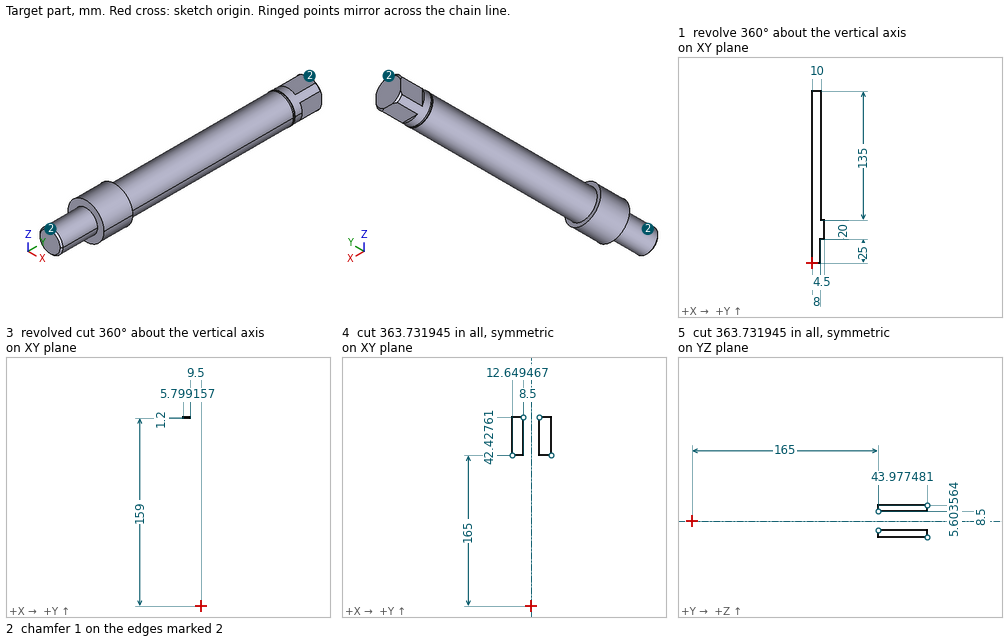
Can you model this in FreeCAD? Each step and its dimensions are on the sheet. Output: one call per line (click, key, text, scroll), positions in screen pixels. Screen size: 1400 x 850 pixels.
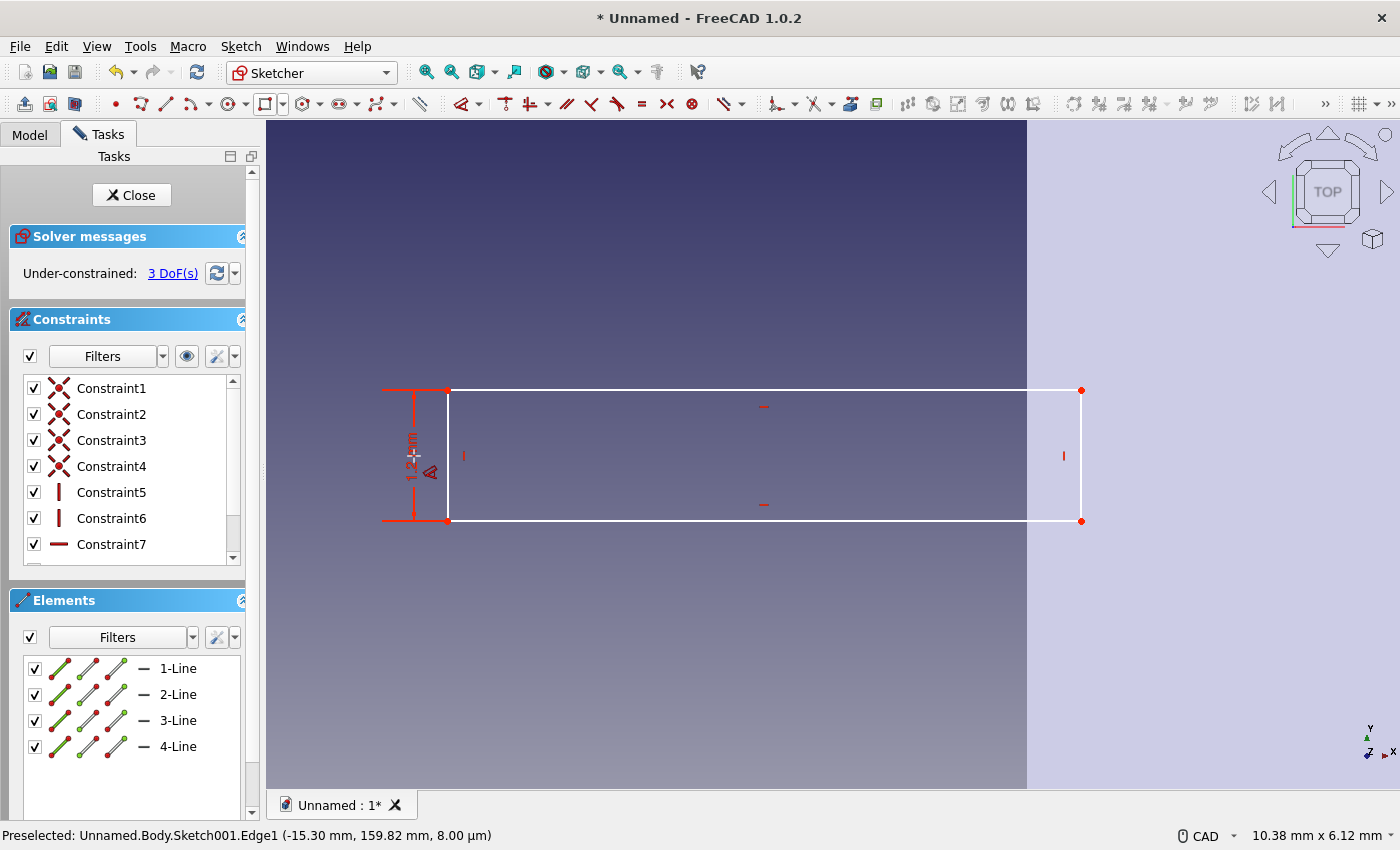
click(448, 521)
click(414, 641)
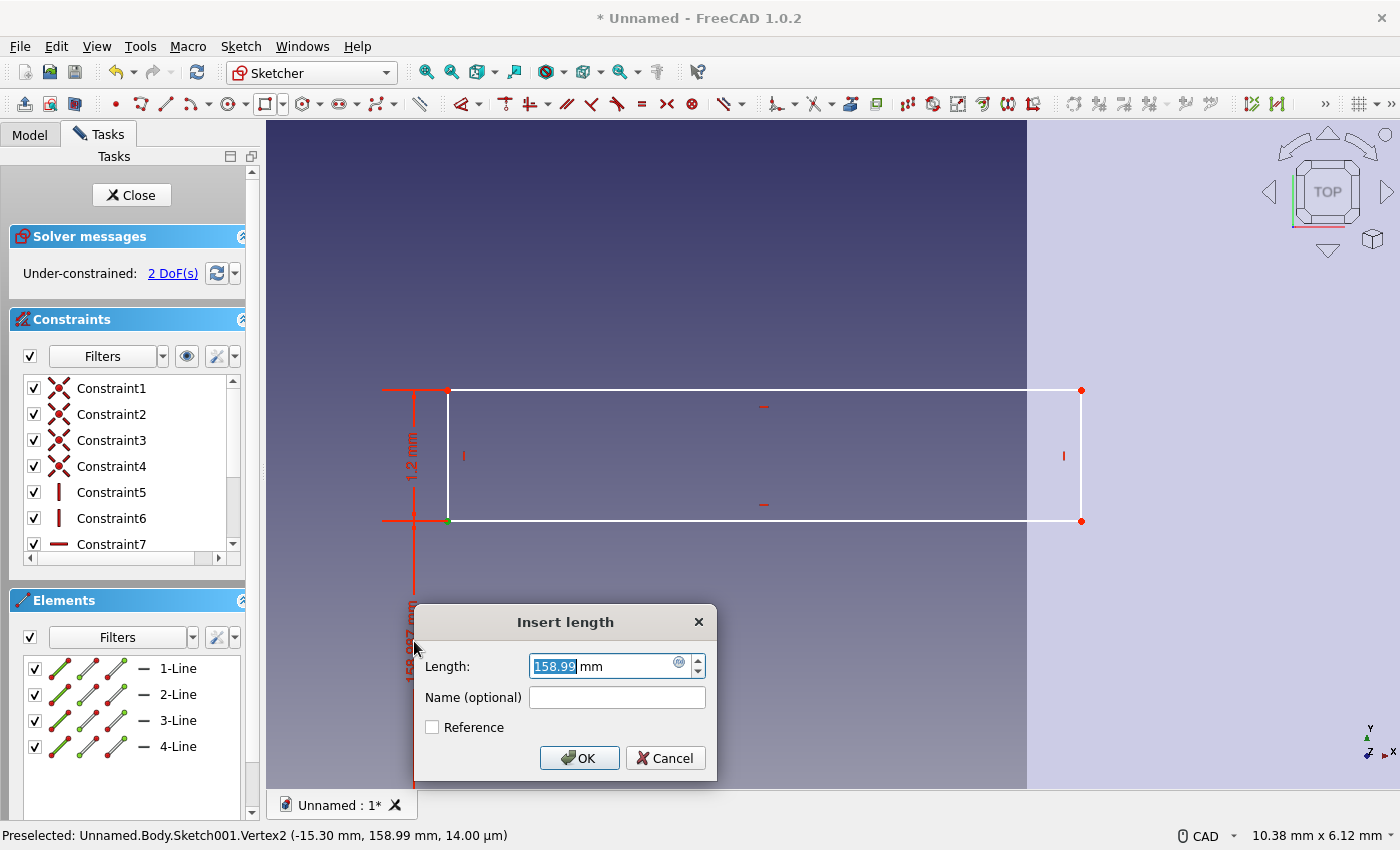
text(159)
key(Return)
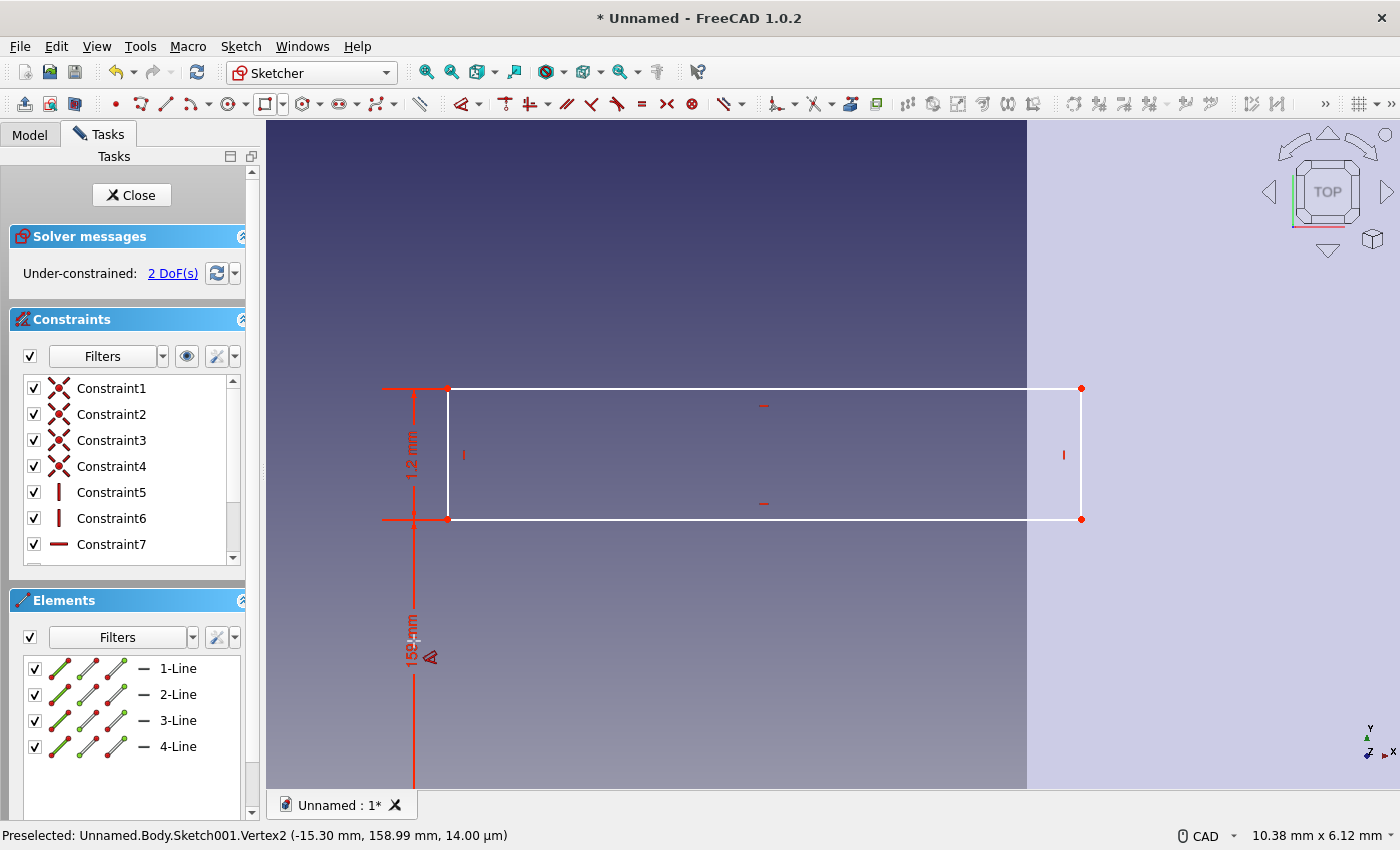
click(1081, 520)
click(1158, 486)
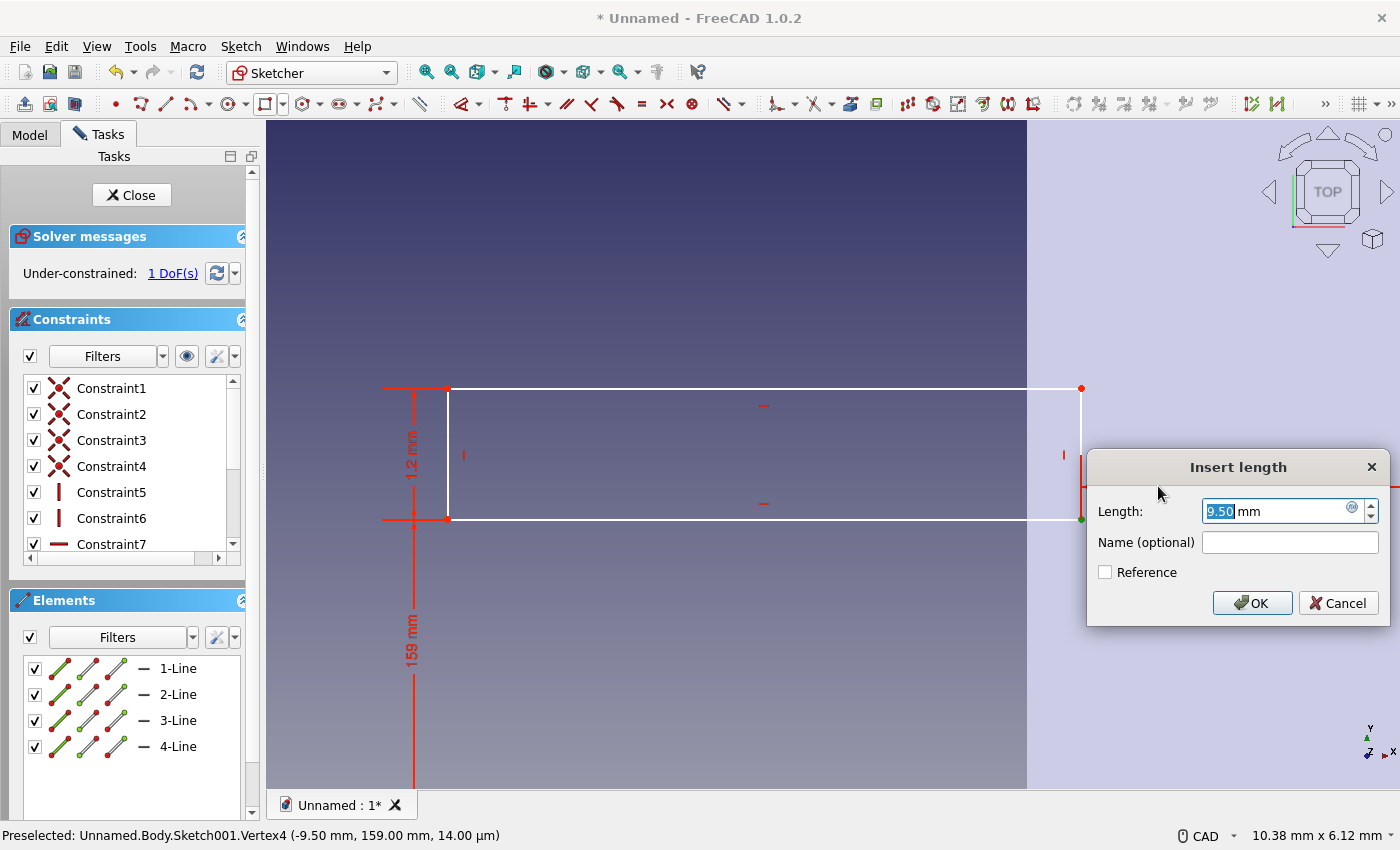
text(9.5)
key(Return)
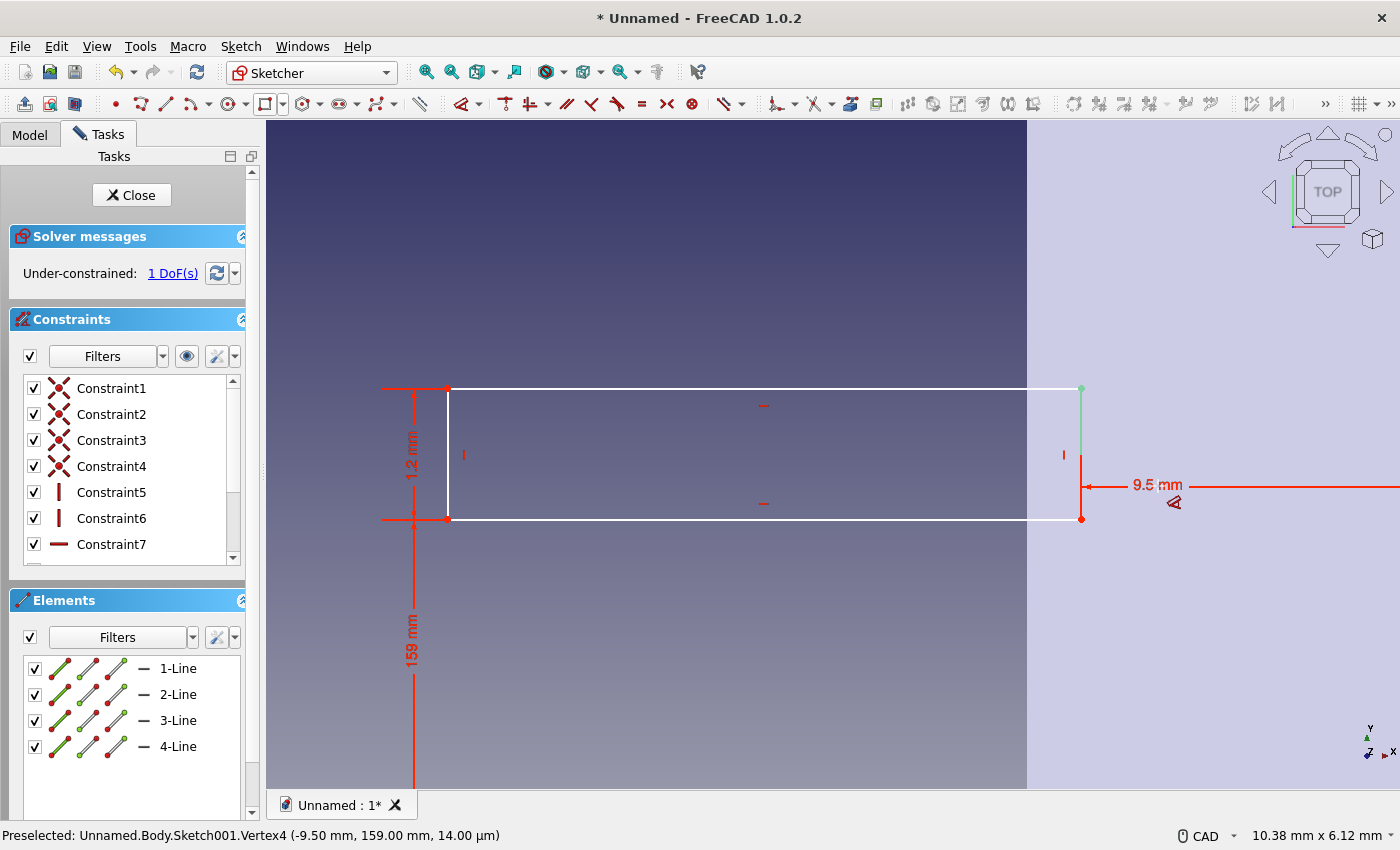
click(638, 520)
click(765, 554)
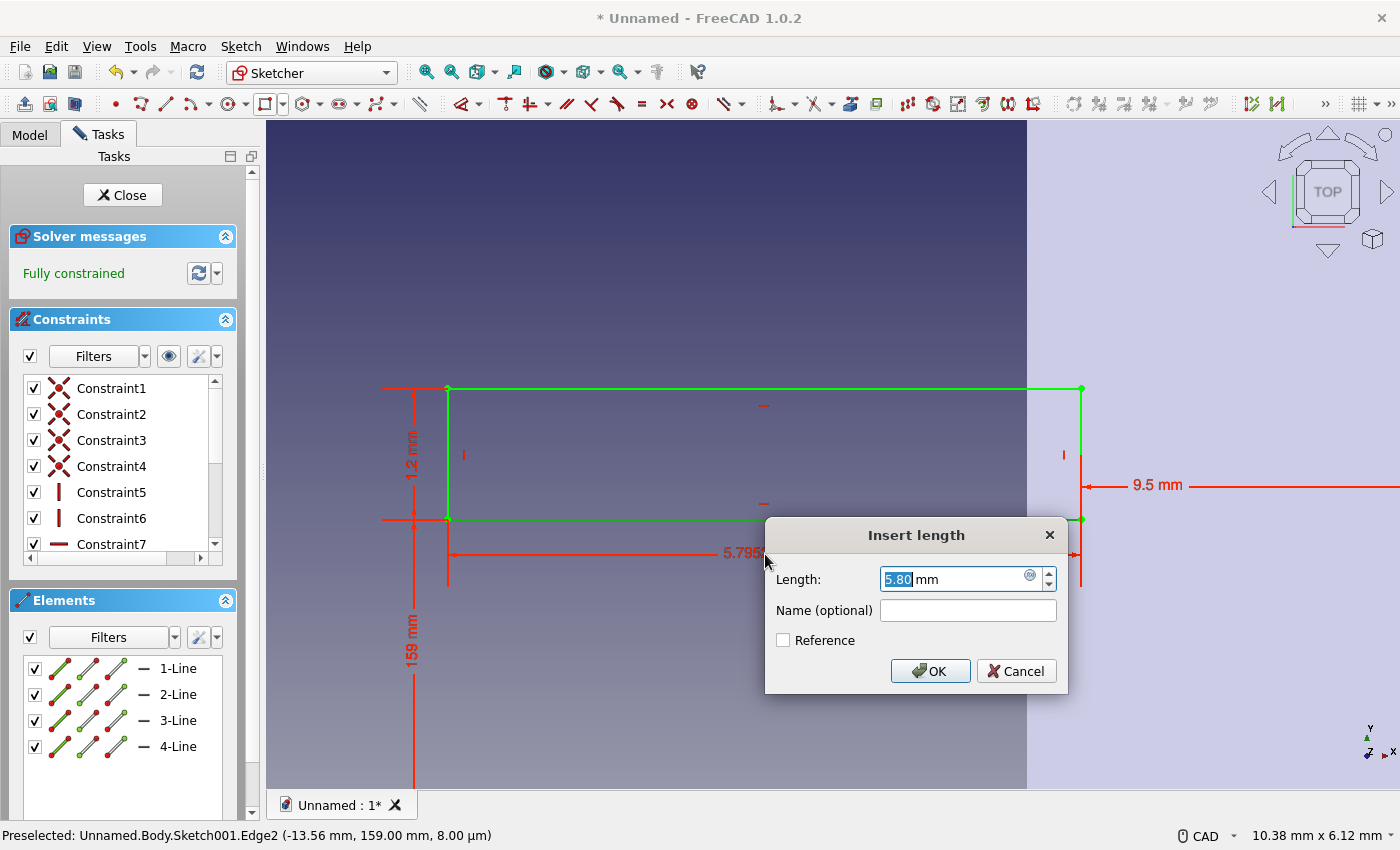
text(5.799157)
key(Return)
key(Escape)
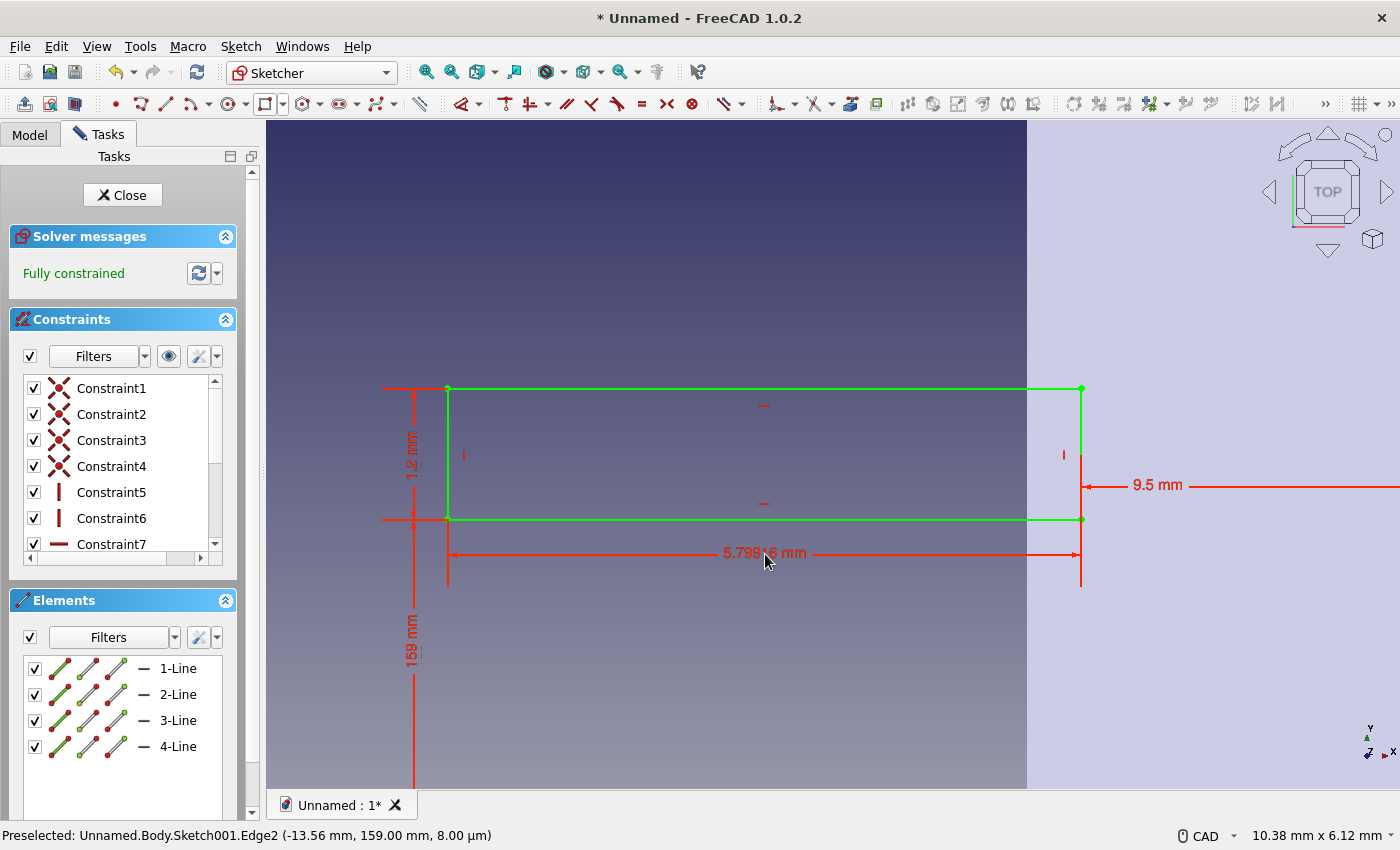
click(123, 195)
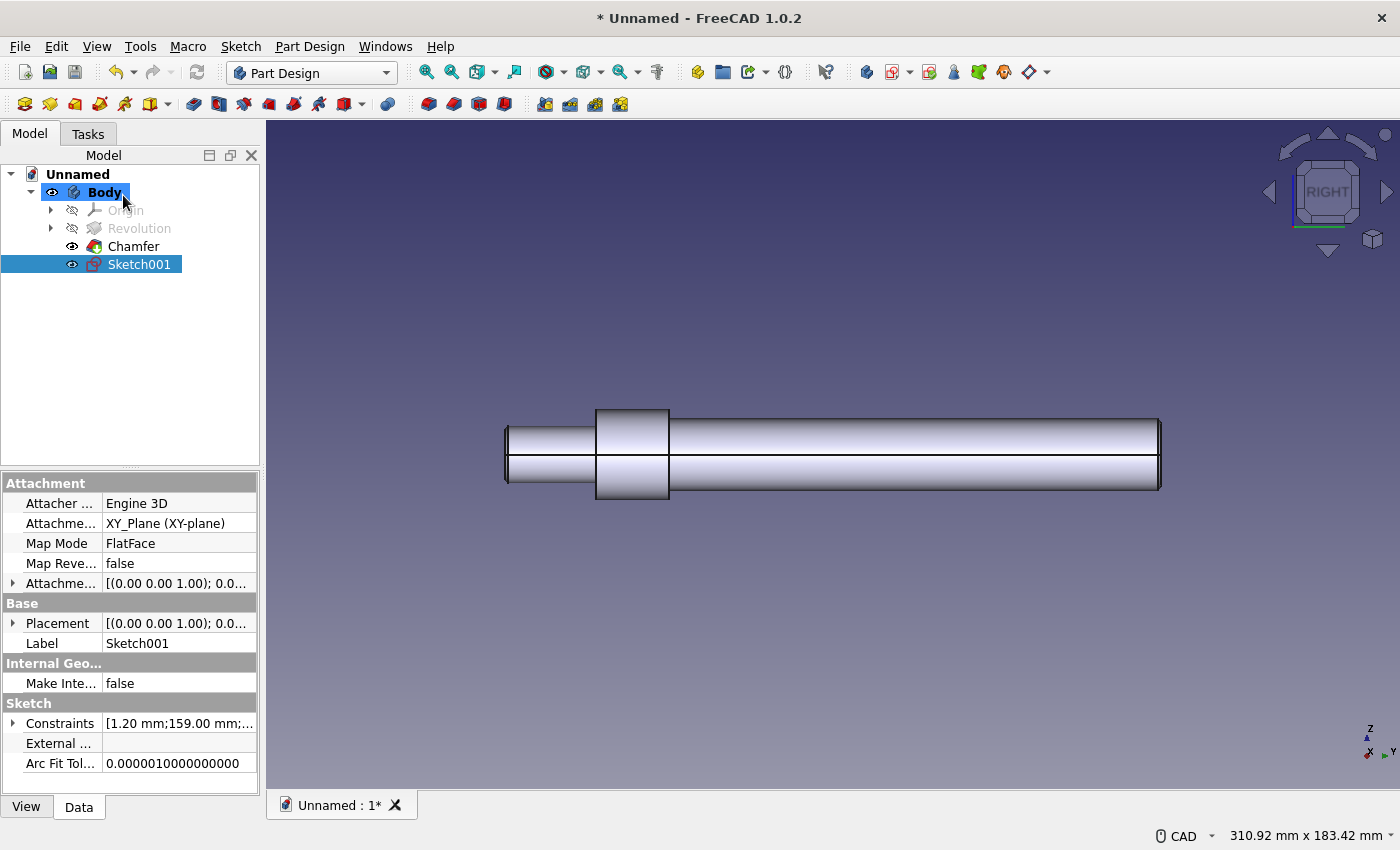
click(244, 104)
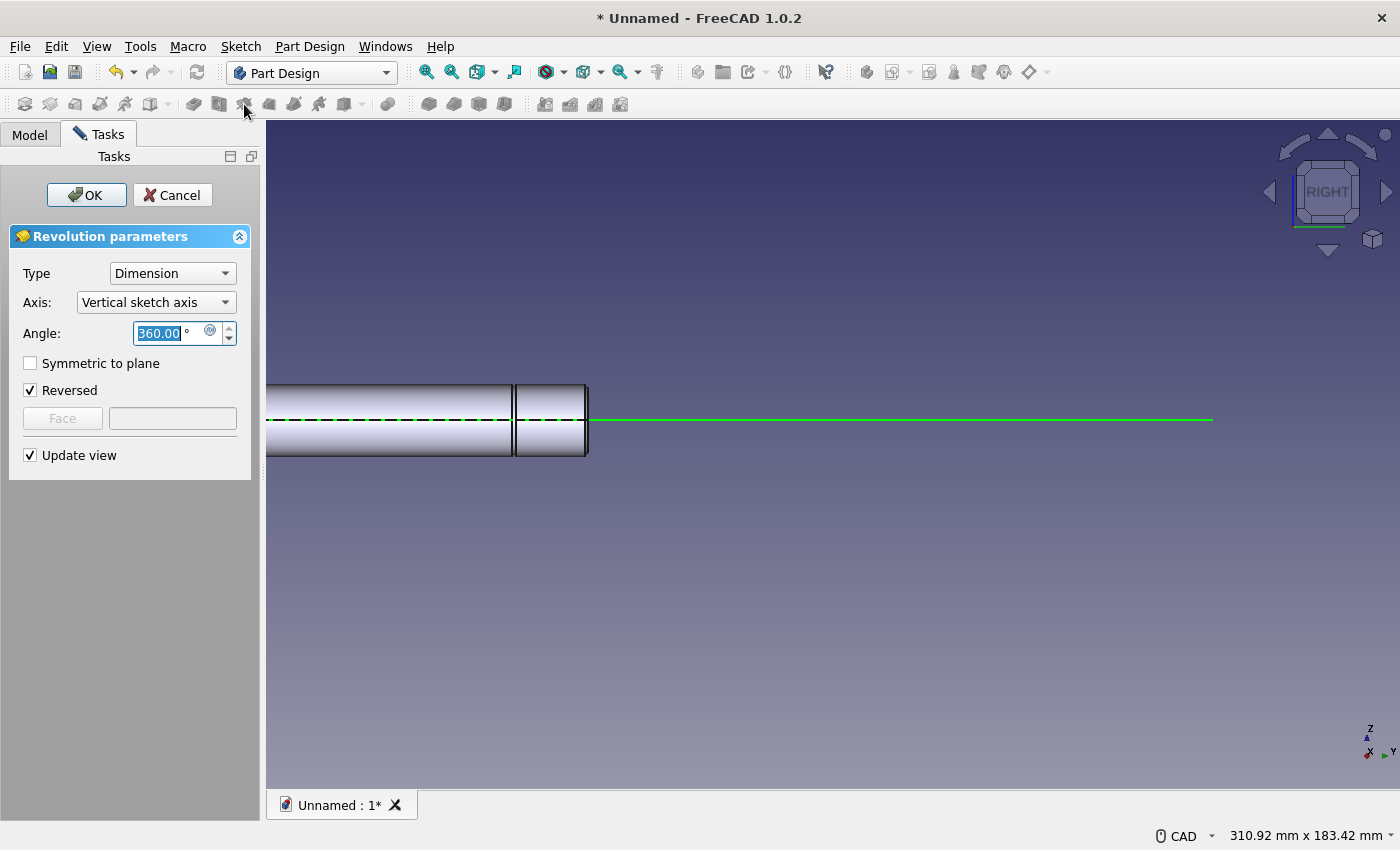
click(87, 195)